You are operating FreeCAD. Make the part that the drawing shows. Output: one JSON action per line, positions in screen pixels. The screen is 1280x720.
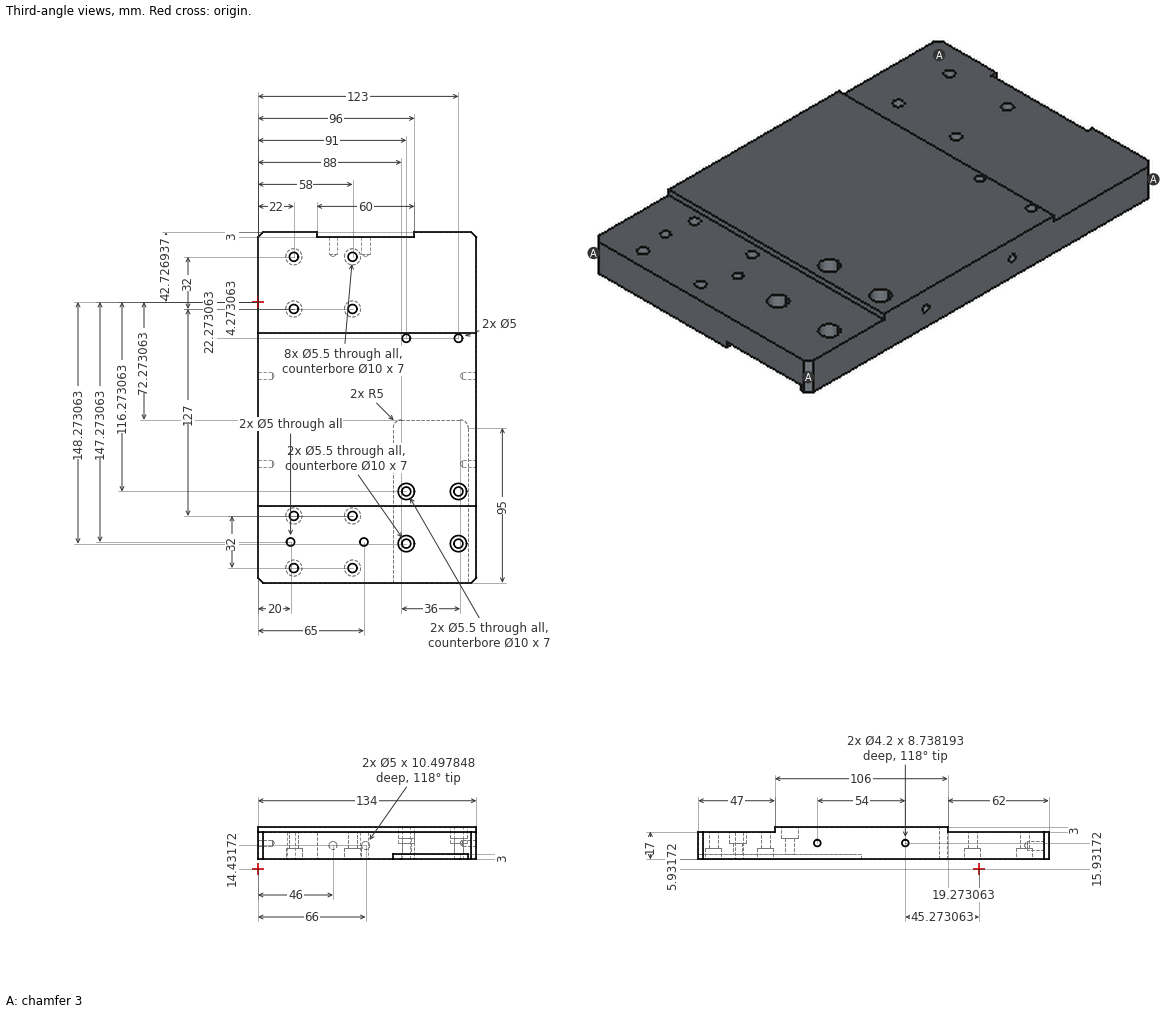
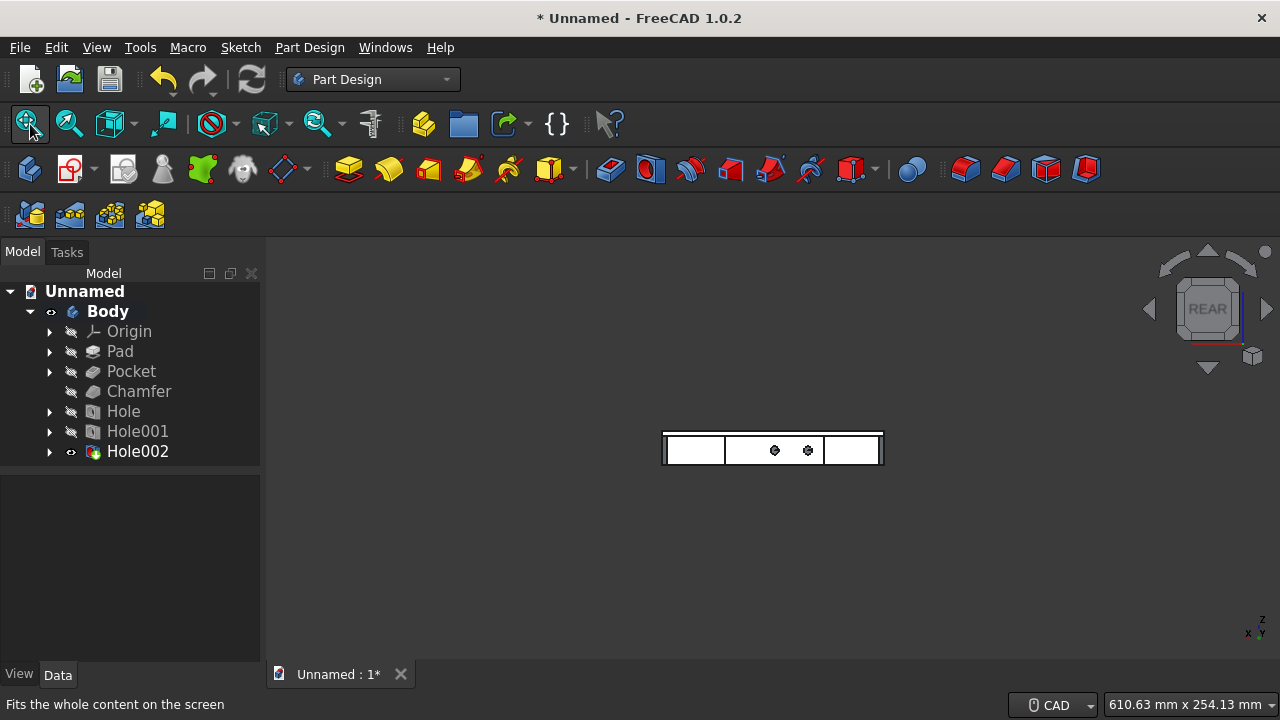
{"action": "key", "text": "5"}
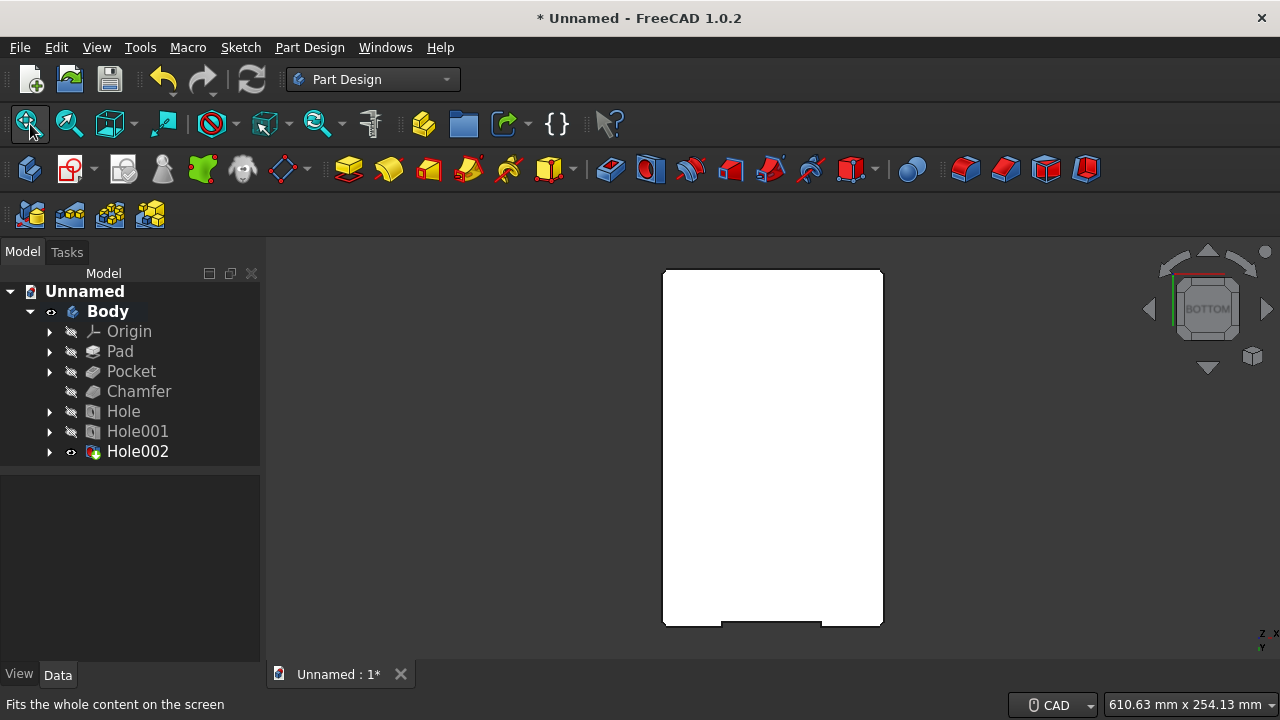
{"action": "left_click", "coordinate": [773, 498]}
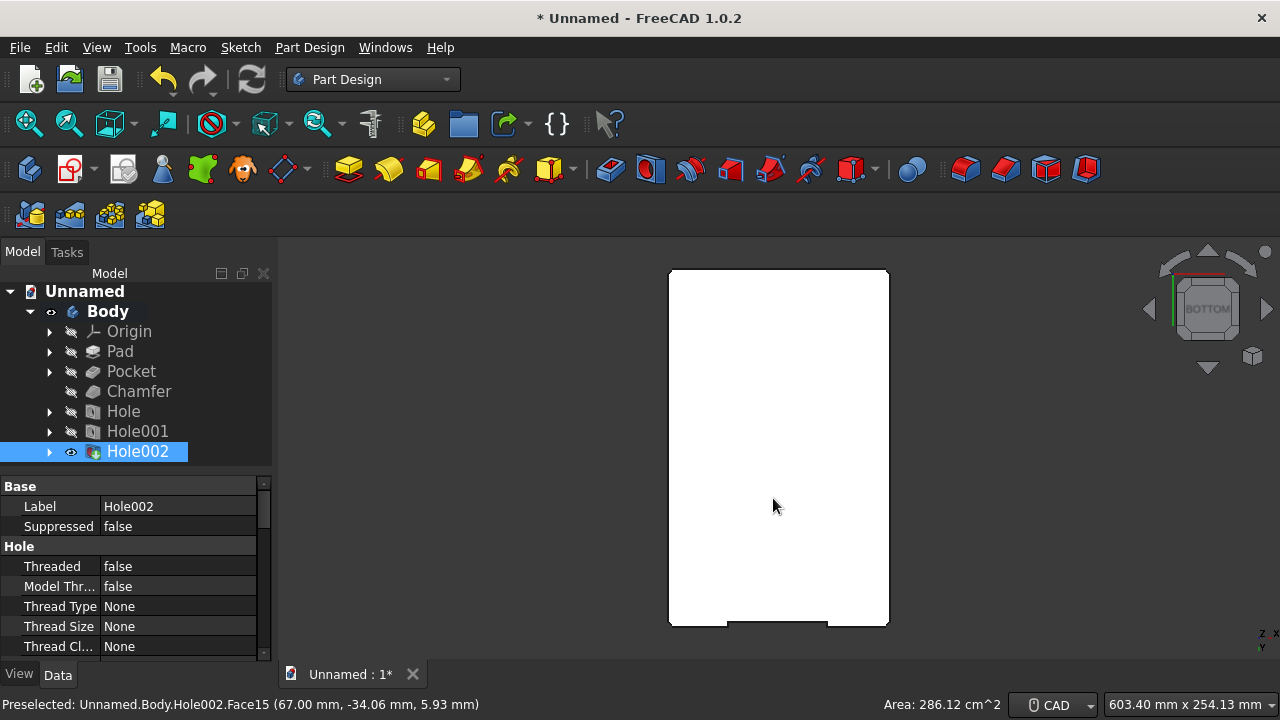
{"action": "left_click", "coordinate": [70, 170]}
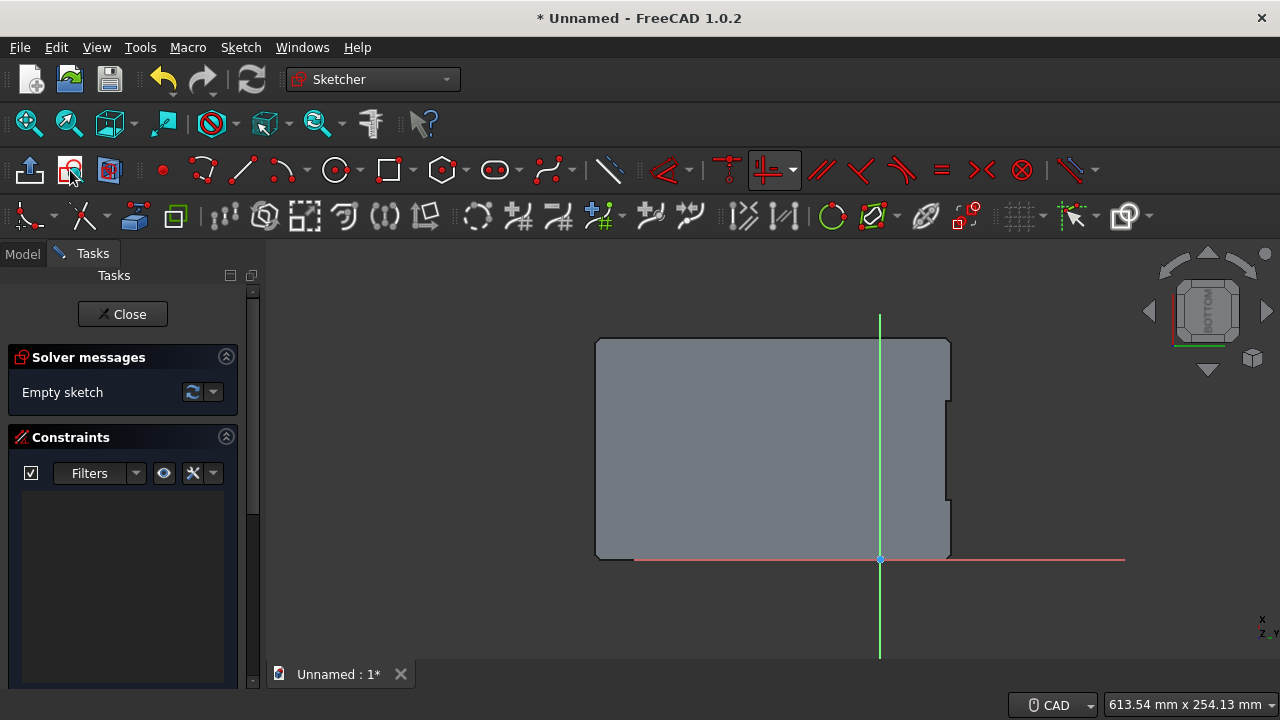
{"action": "scroll", "coordinate": [889, 361], "scroll_direction": "up", "scroll_amount": 7}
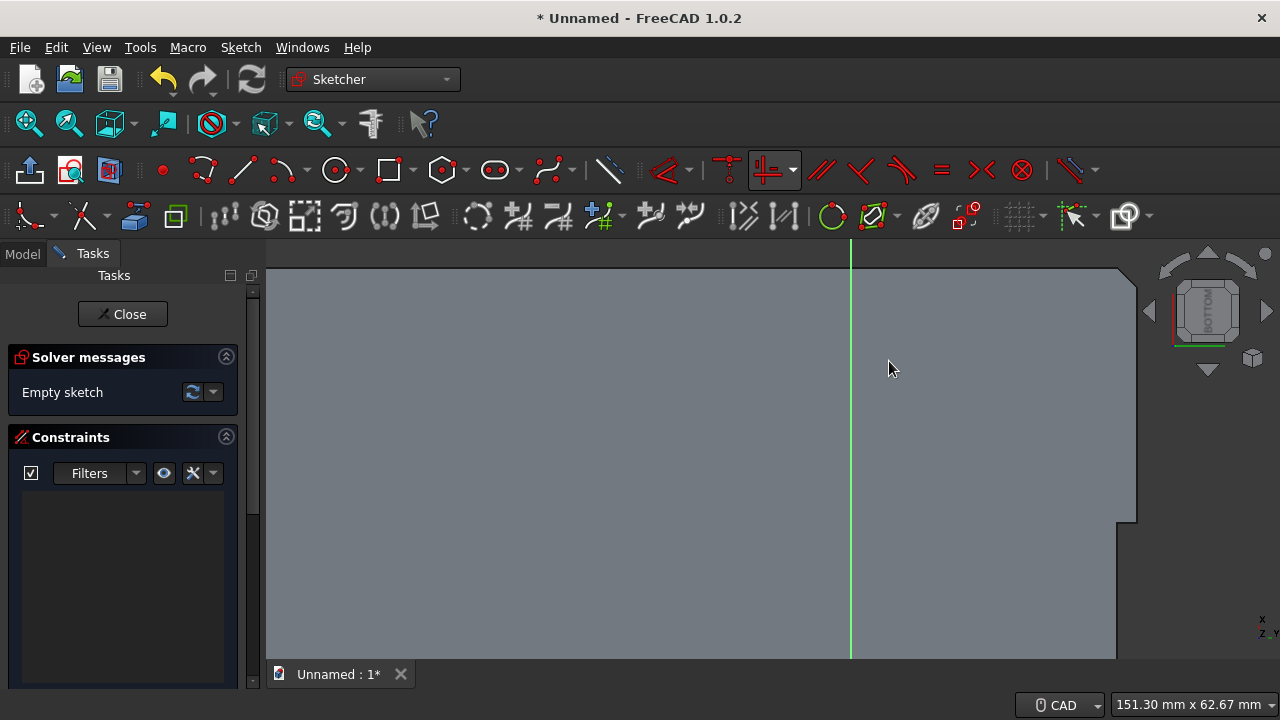
{"action": "left_click", "coordinate": [336, 170]}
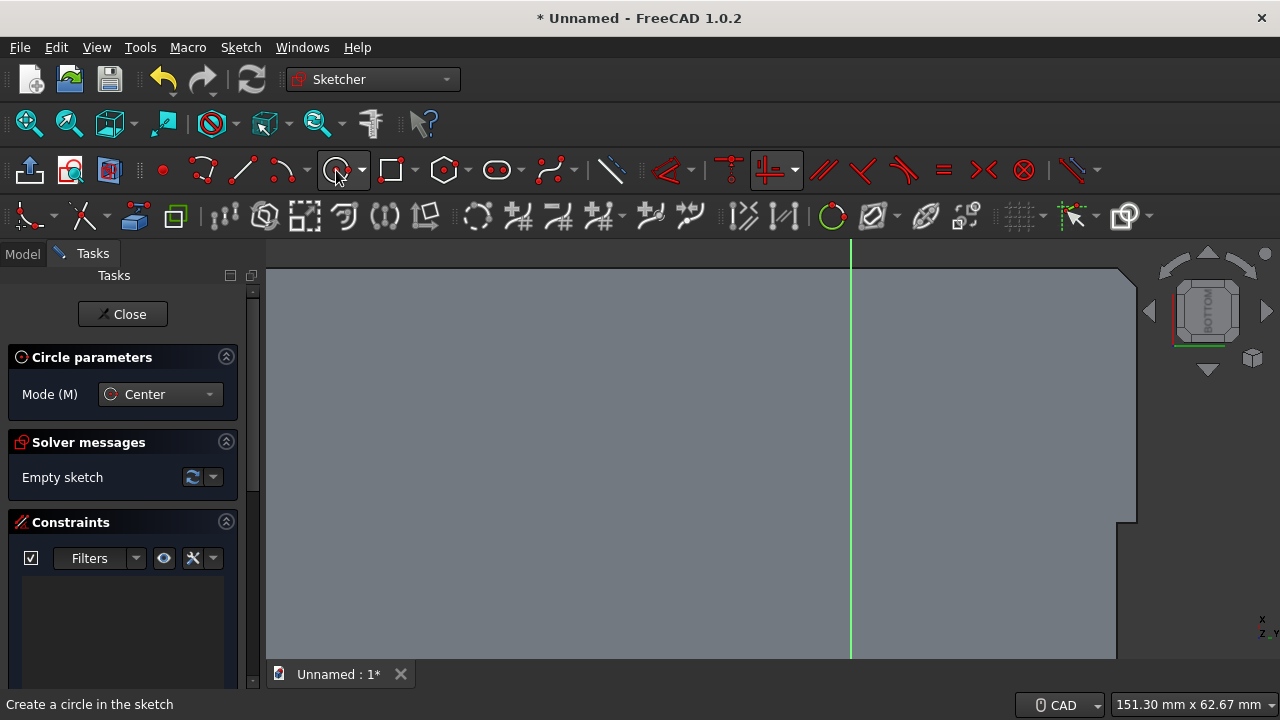
{"action": "scroll", "coordinate": [702, 342], "scroll_direction": "up", "scroll_amount": 2}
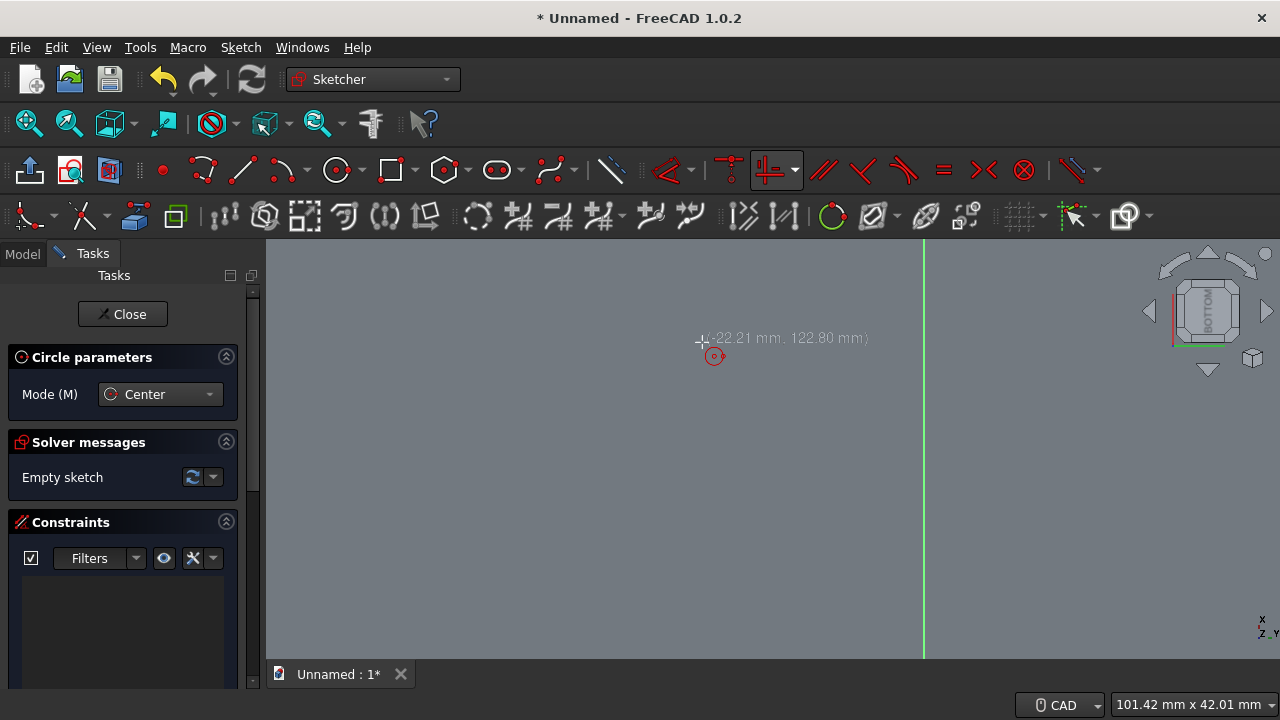
{"action": "left_click", "coordinate": [701, 341]}
{"action": "mouse_move", "coordinate": [719, 324]}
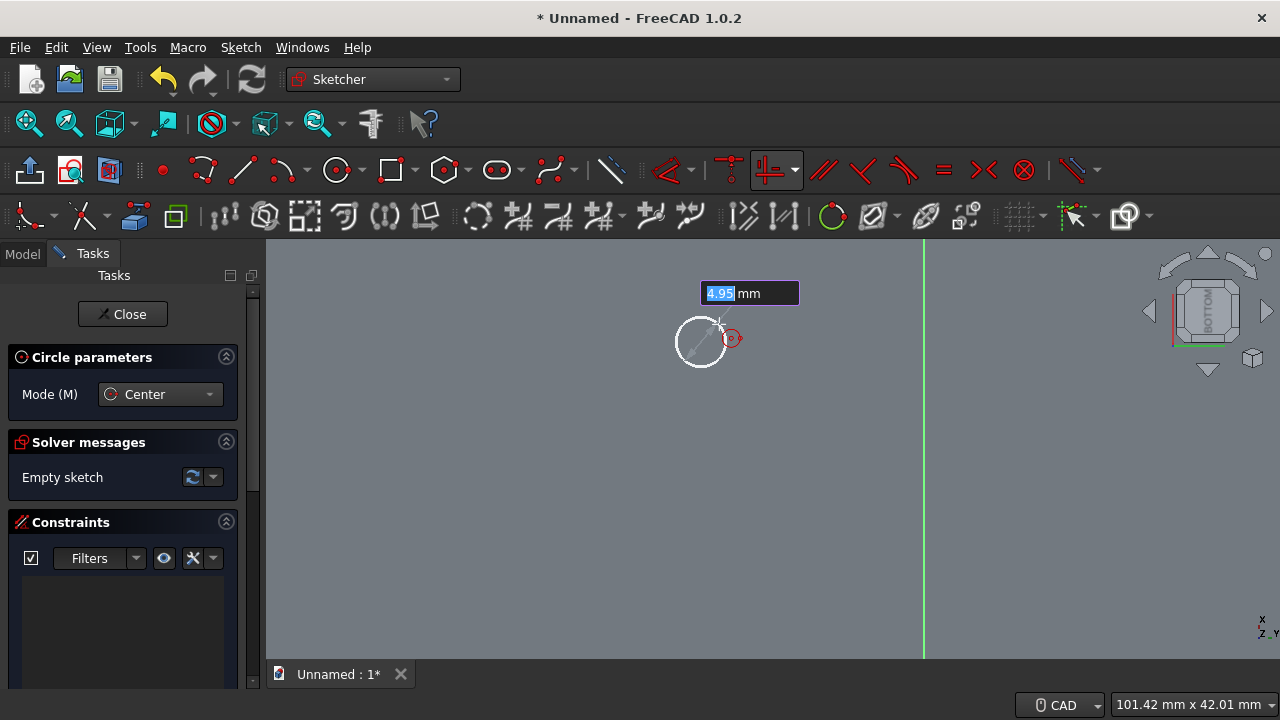
{"action": "type", "text": "5"}
{"action": "key", "text": "Return"}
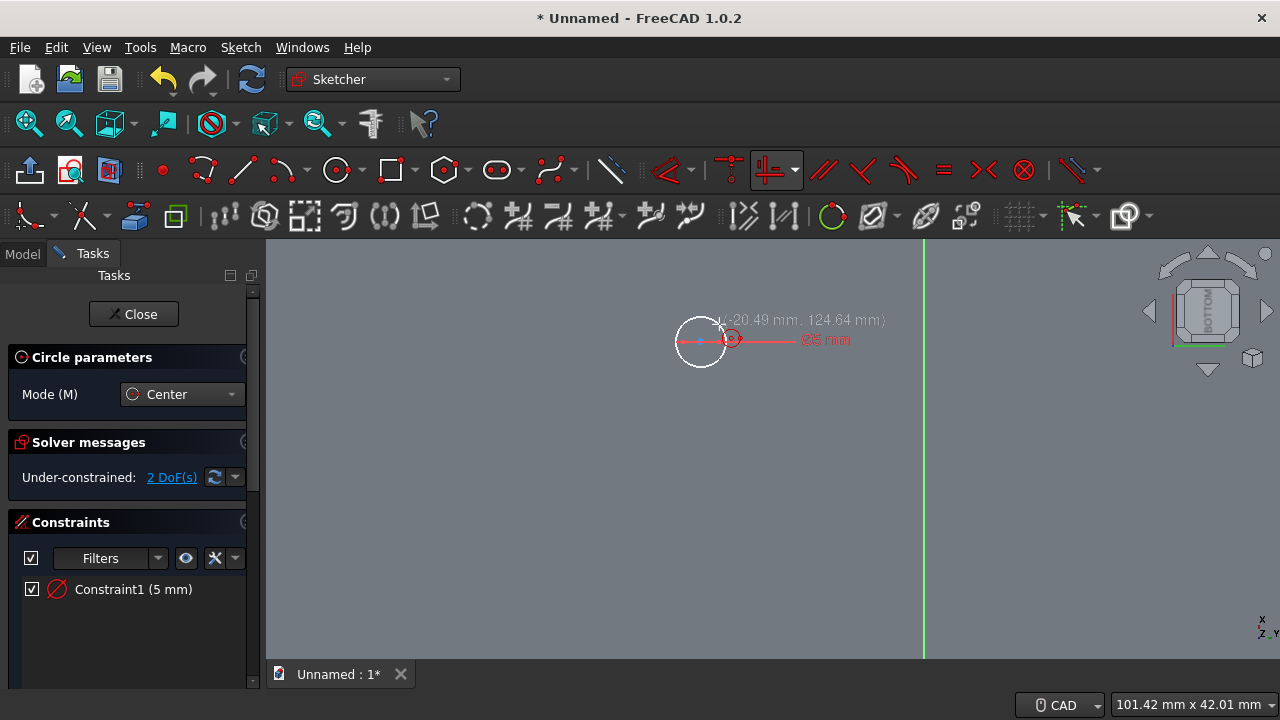
{"action": "scroll", "coordinate": [711, 343], "scroll_direction": "down", "scroll_amount": 2}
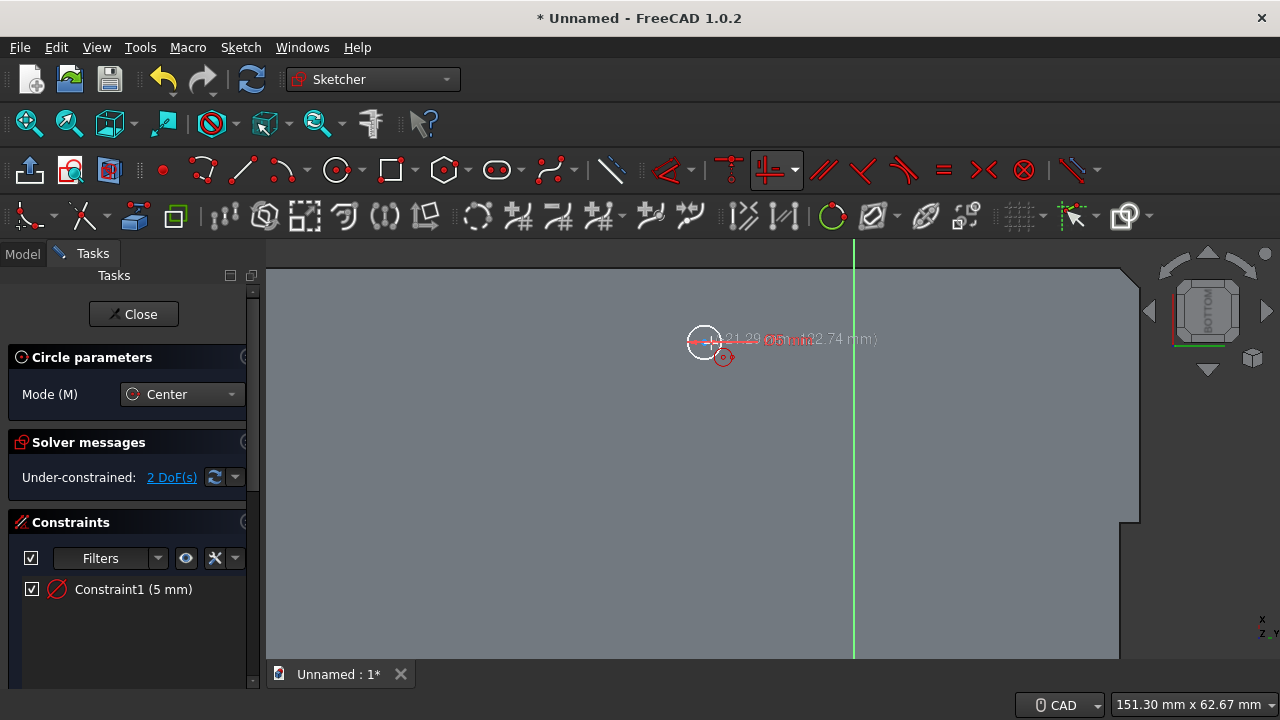
{"action": "scroll", "coordinate": [705, 556], "scroll_direction": "up", "scroll_amount": 2}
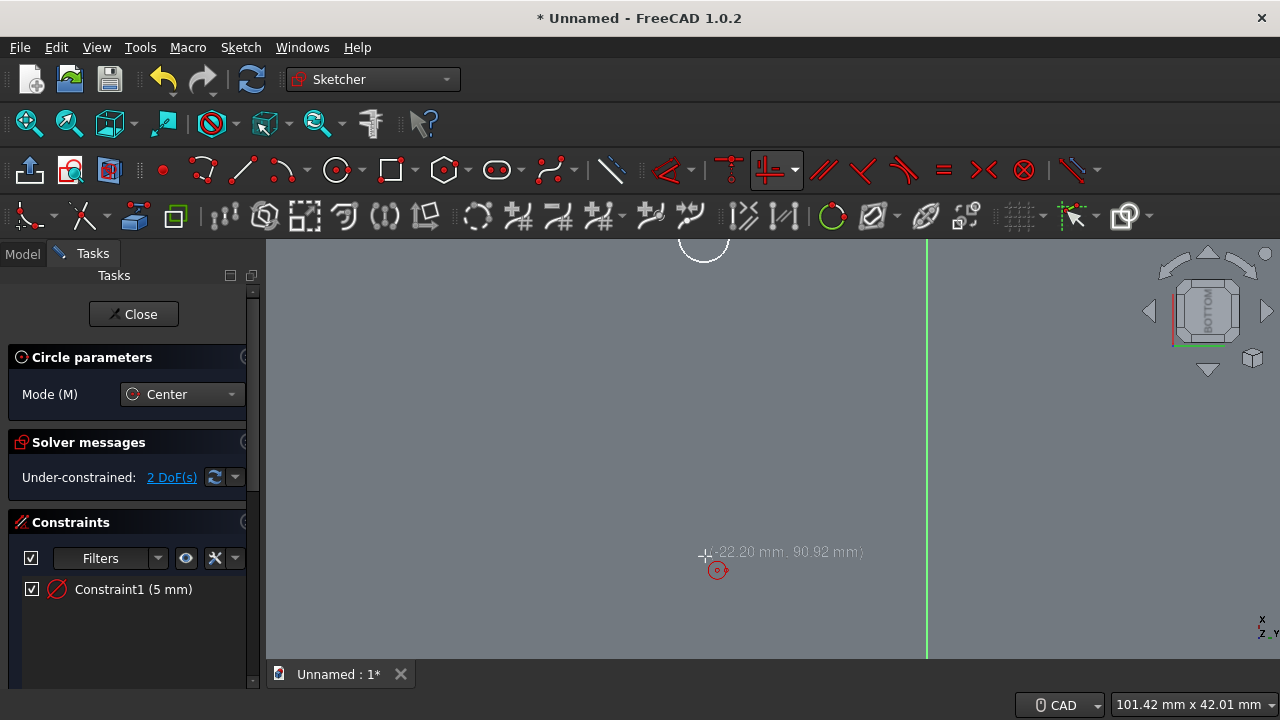
{"action": "left_click", "coordinate": [704, 556]}
{"action": "mouse_move", "coordinate": [722, 539]}